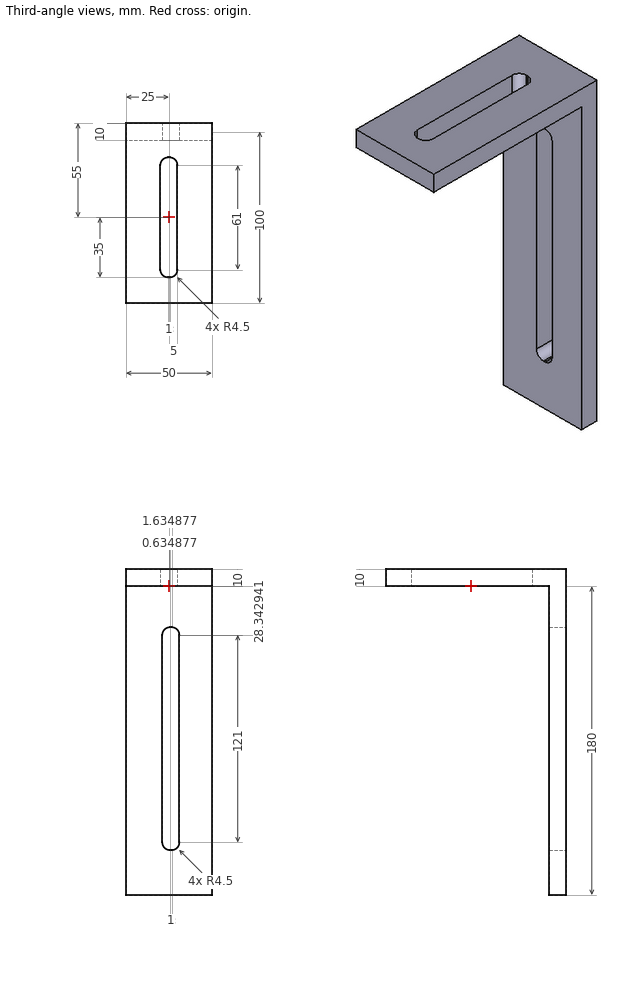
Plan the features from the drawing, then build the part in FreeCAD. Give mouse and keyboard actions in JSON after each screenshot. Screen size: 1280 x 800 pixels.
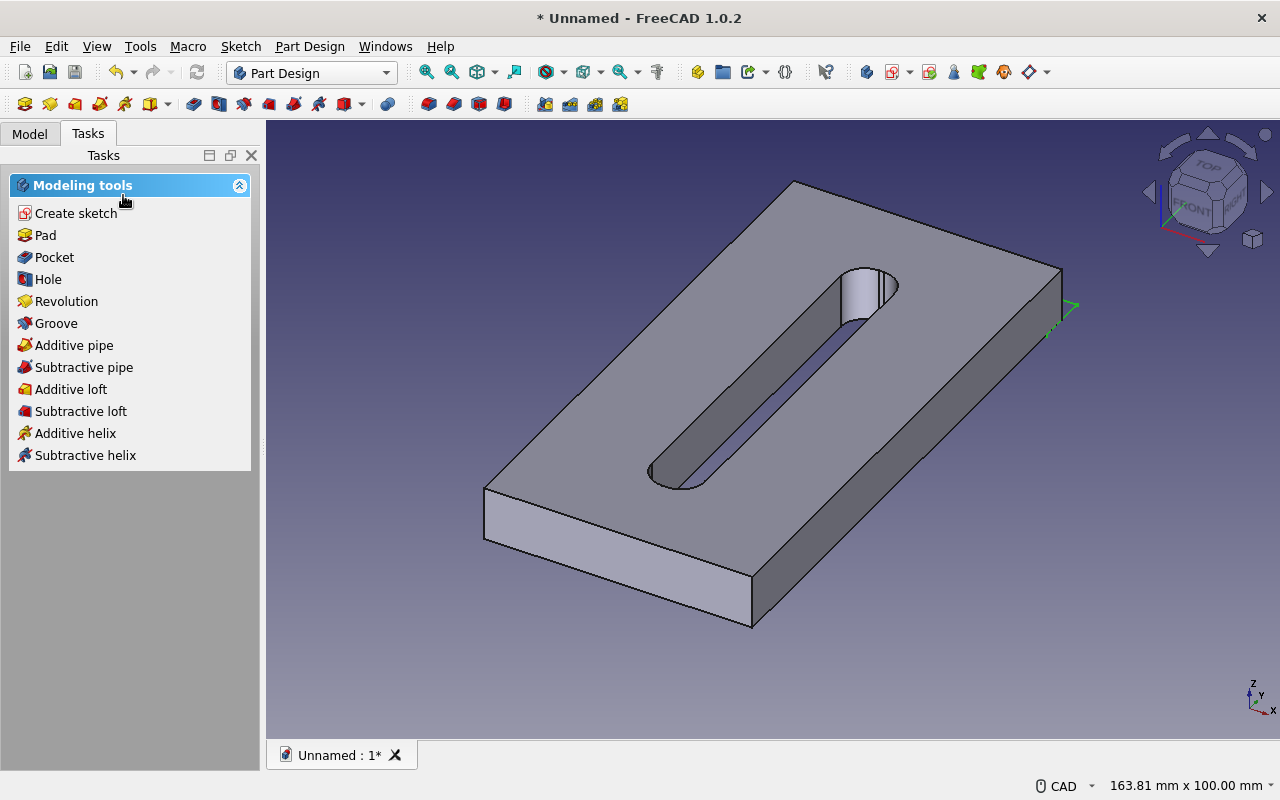
{"action": "left_click", "coordinate": [25, 104]}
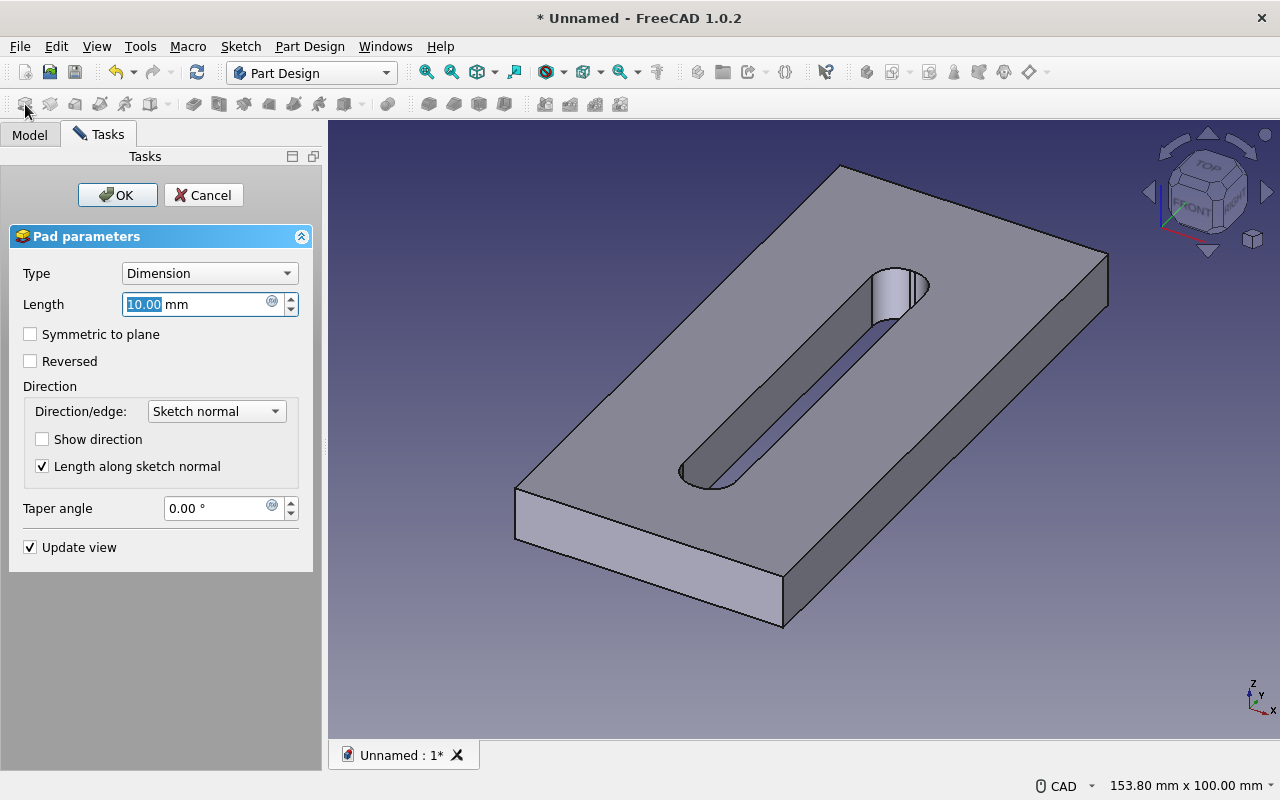
{"action": "left_click", "coordinate": [210, 274]}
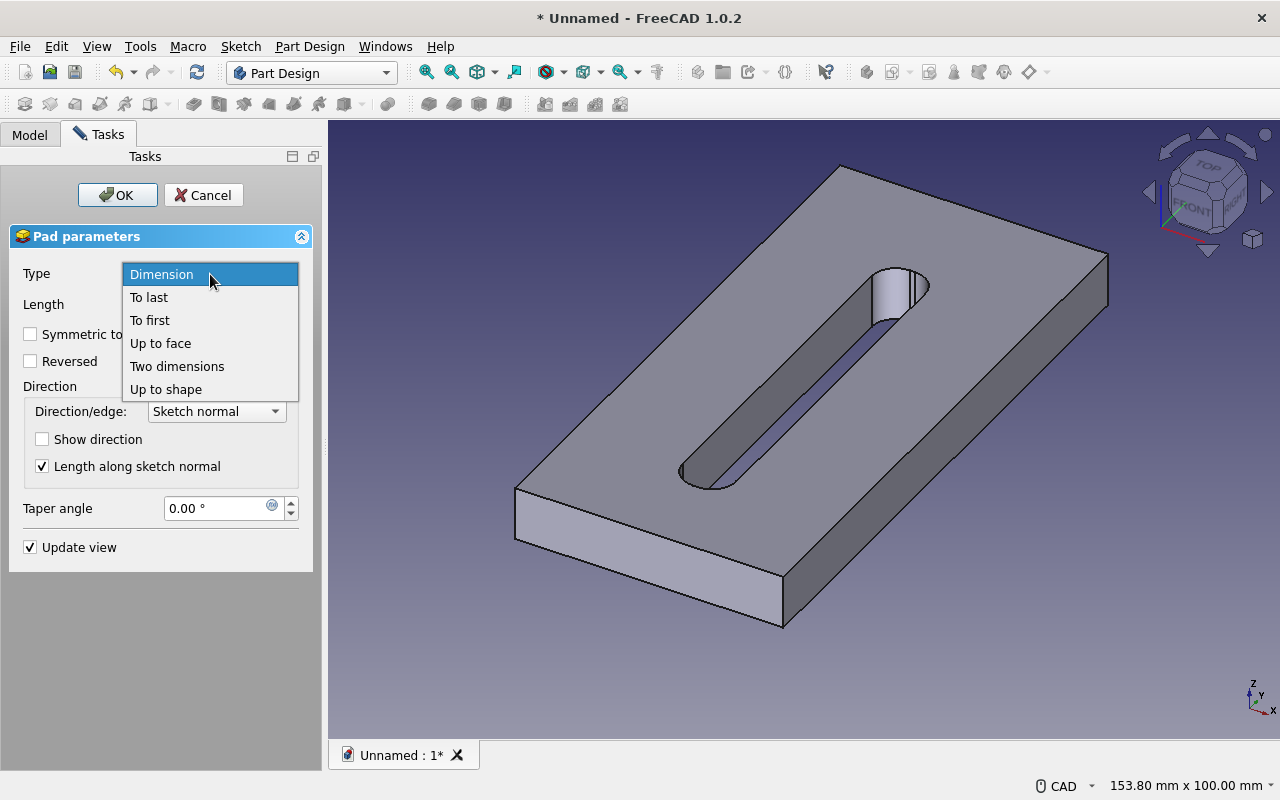
{"action": "left_click", "coordinate": [208, 366]}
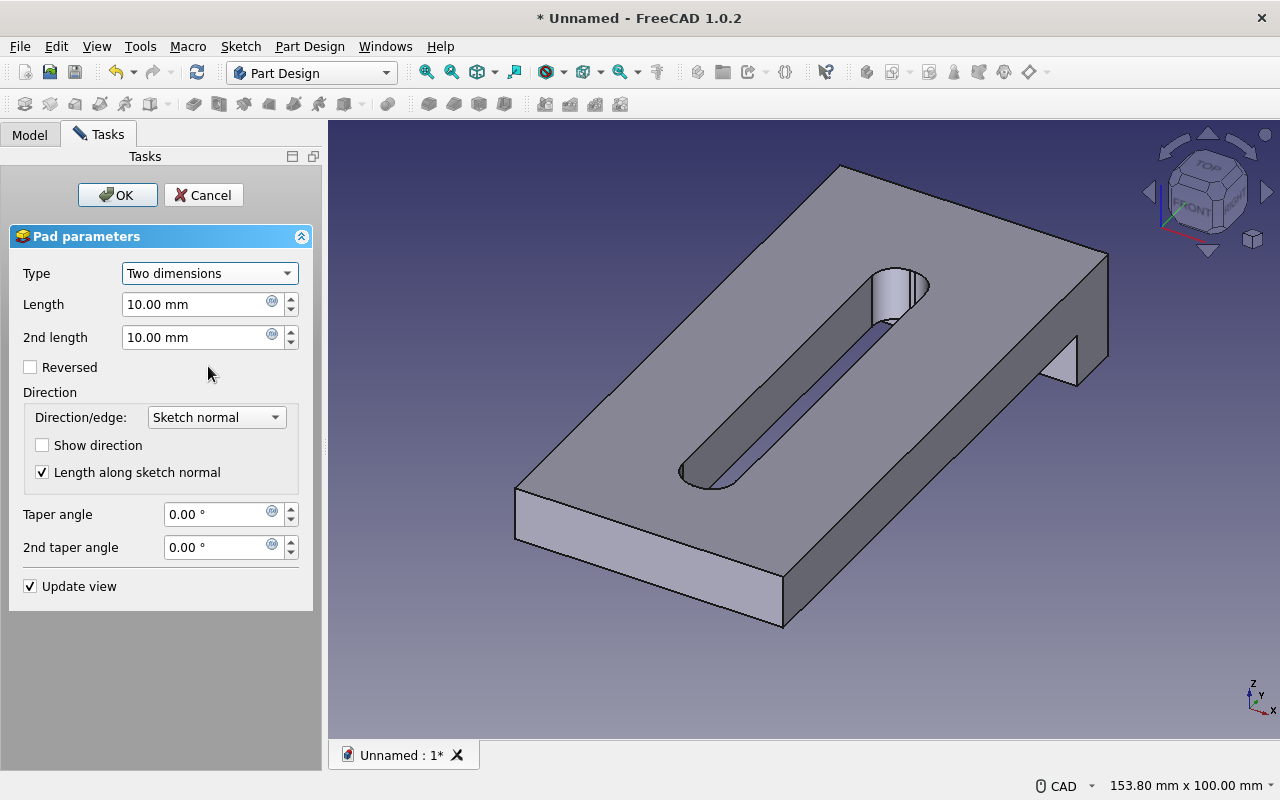
{"action": "triple_click", "coordinate": [204, 304]}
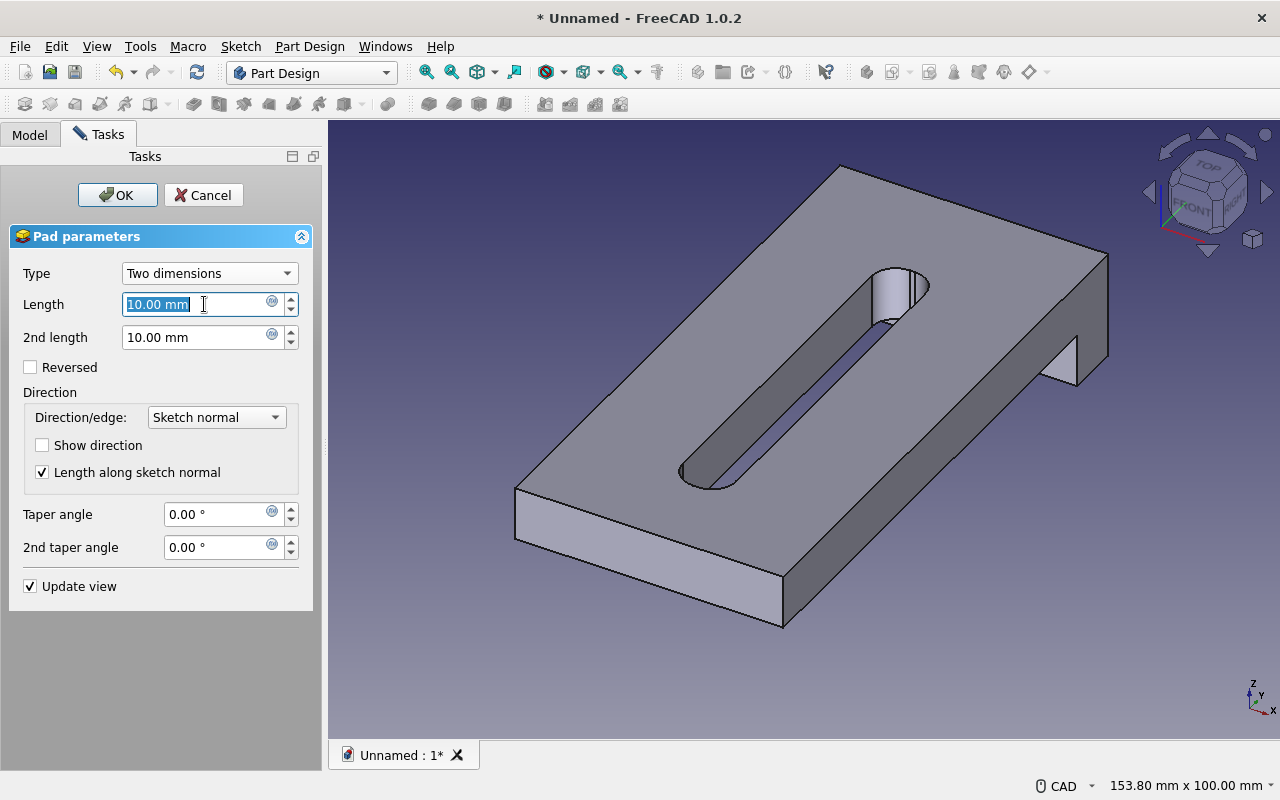
{"action": "type", "text": "180"}
{"action": "key", "text": "Tab"}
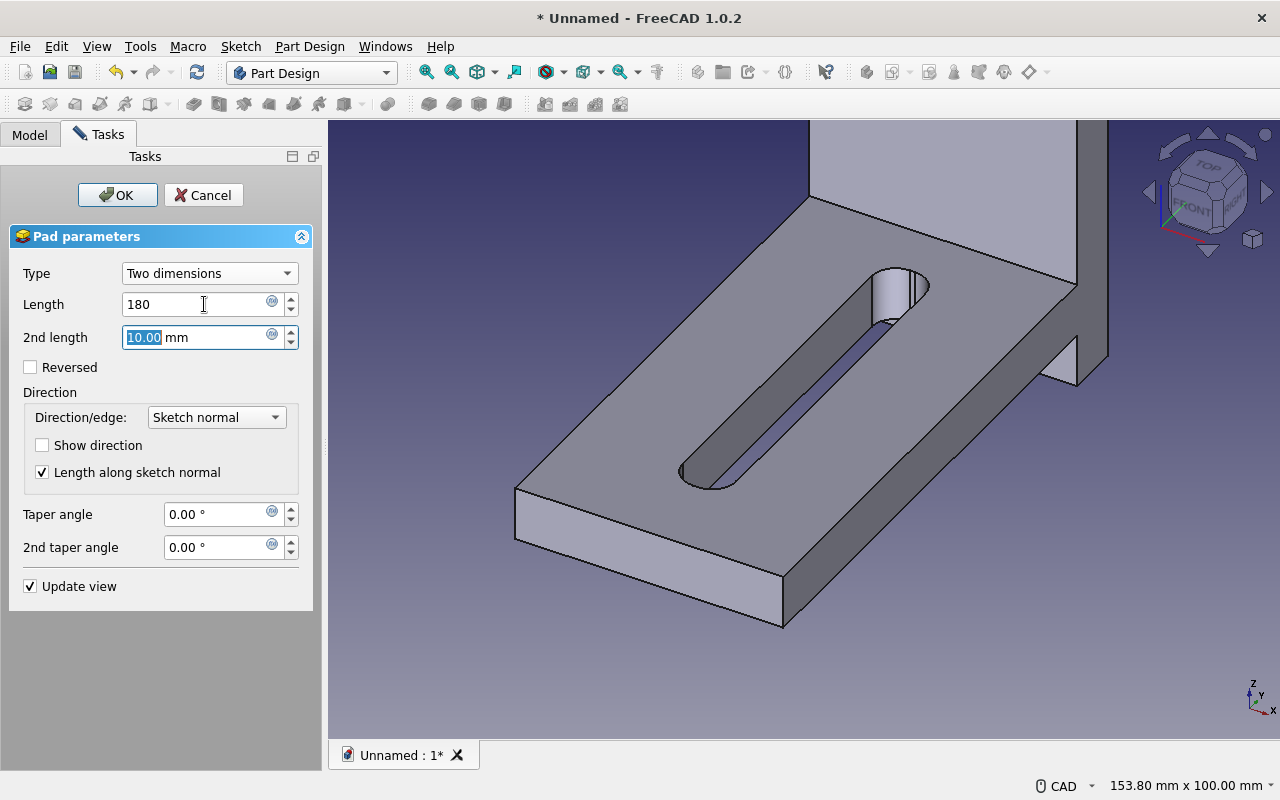
{"action": "type", "text": "10"}
{"action": "key", "text": "Tab"}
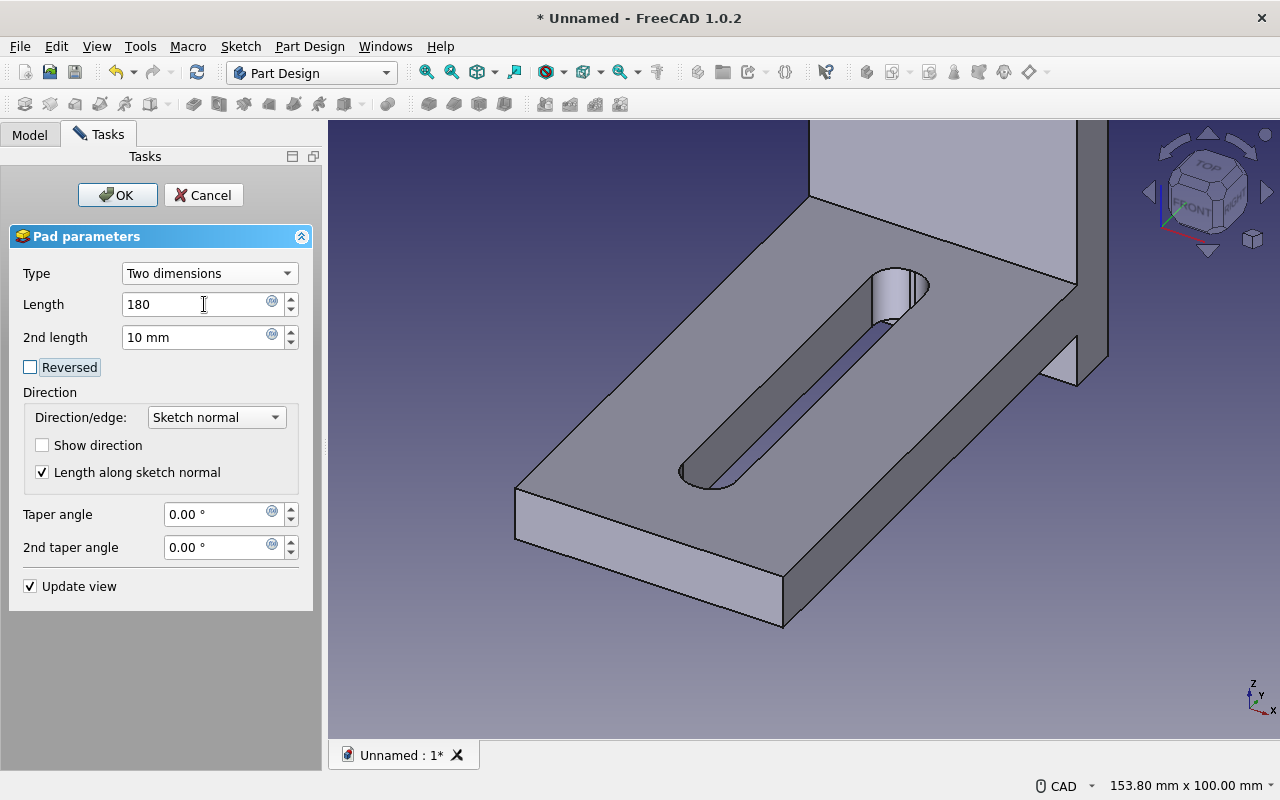
{"action": "left_click", "coordinate": [31, 367]}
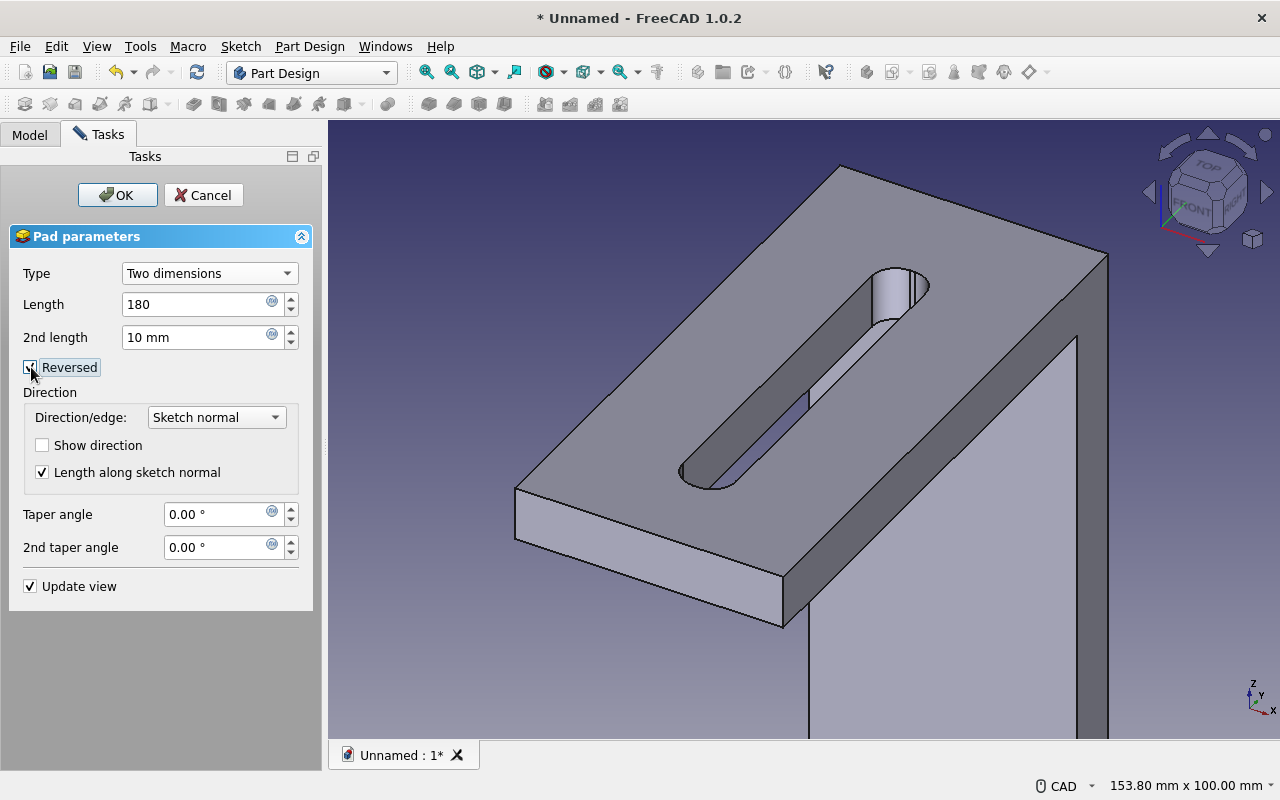
{"action": "left_click", "coordinate": [118, 195]}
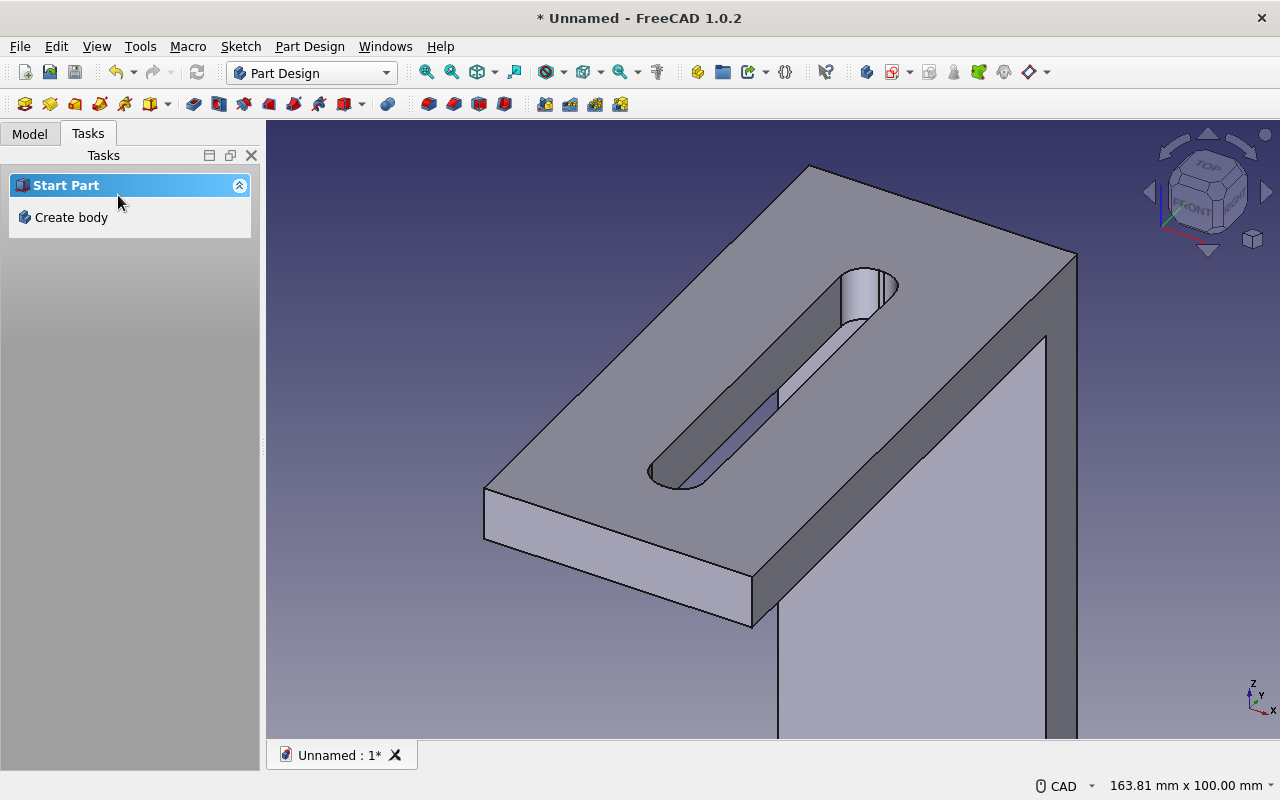
{"action": "left_click", "coordinate": [427, 72]}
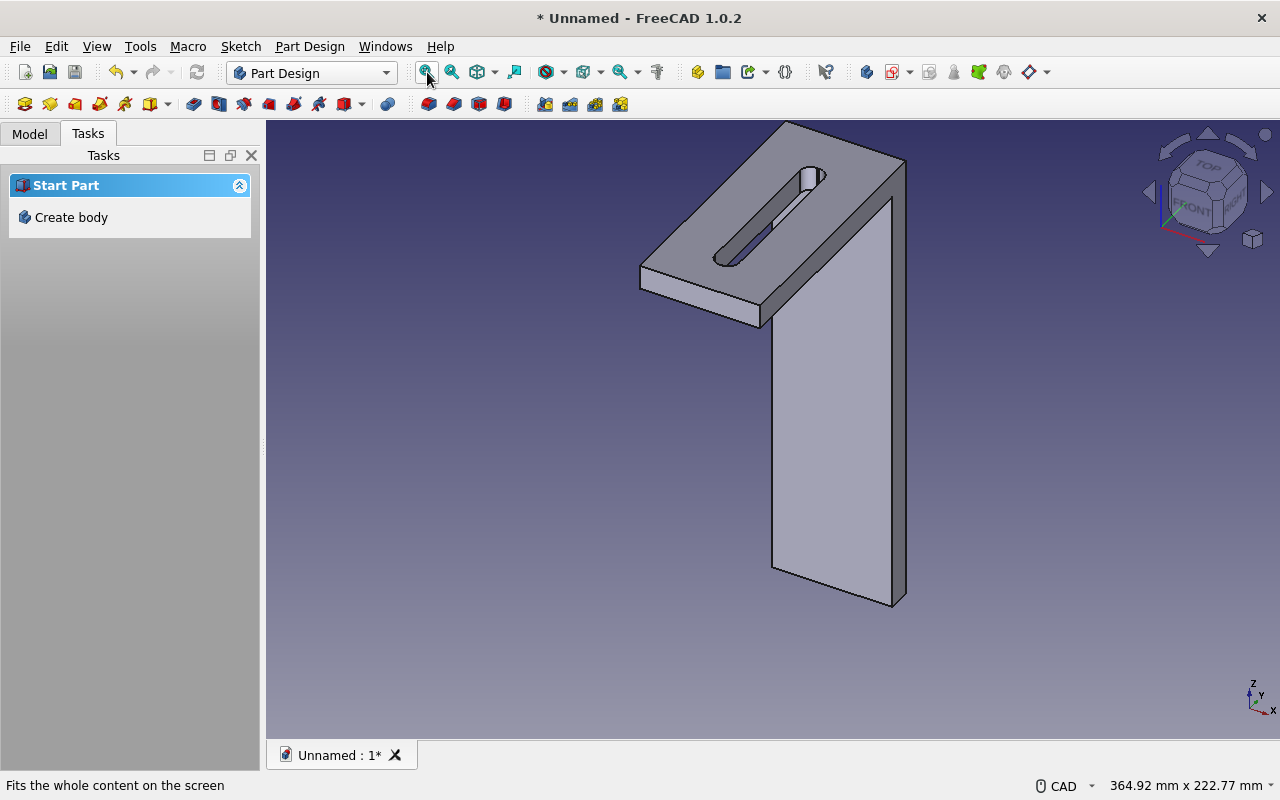
{"action": "left_click", "coordinate": [832, 323]}